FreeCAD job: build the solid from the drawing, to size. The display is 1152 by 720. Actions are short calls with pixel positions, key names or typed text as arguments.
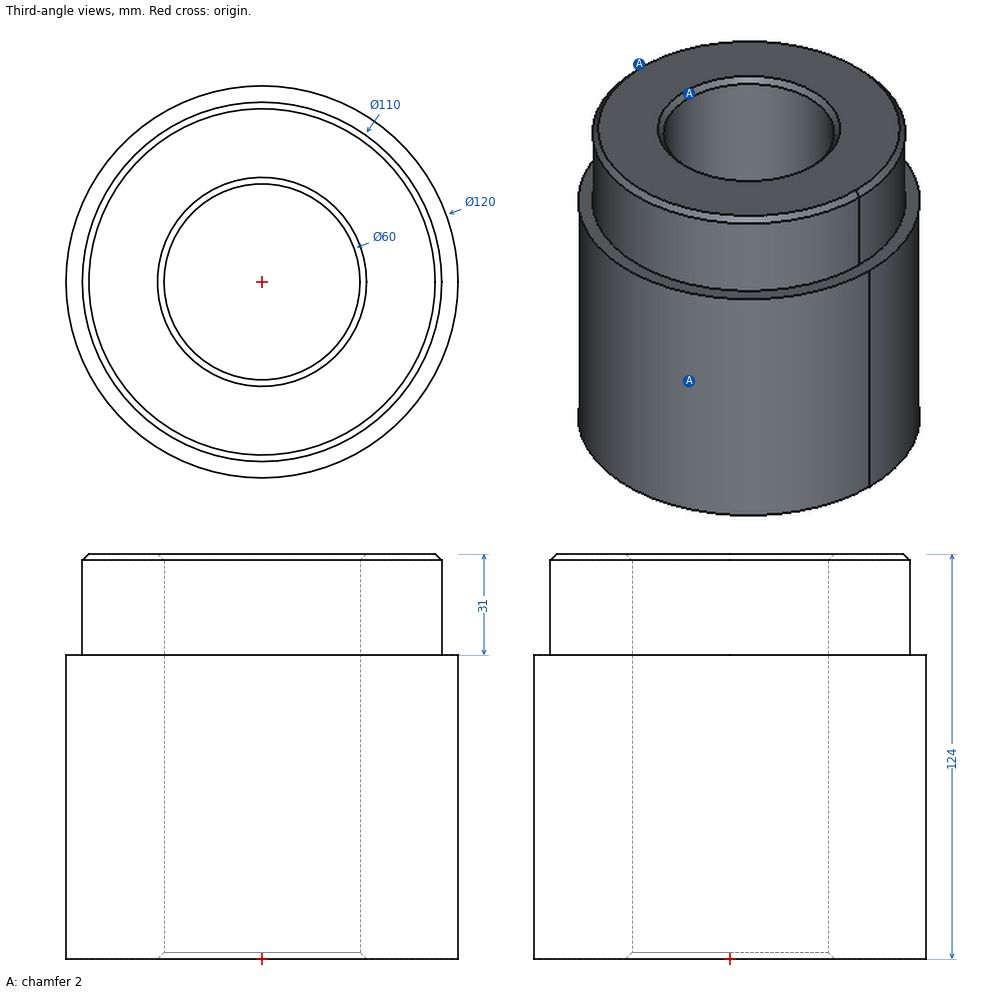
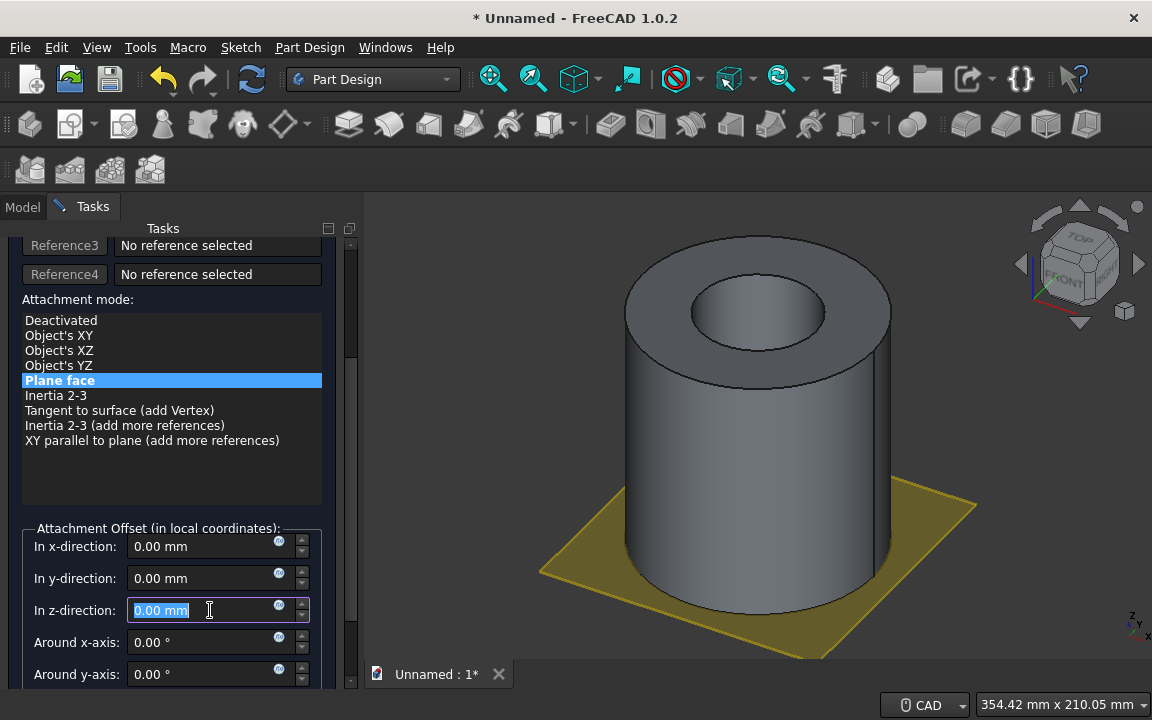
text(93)
key(Tab)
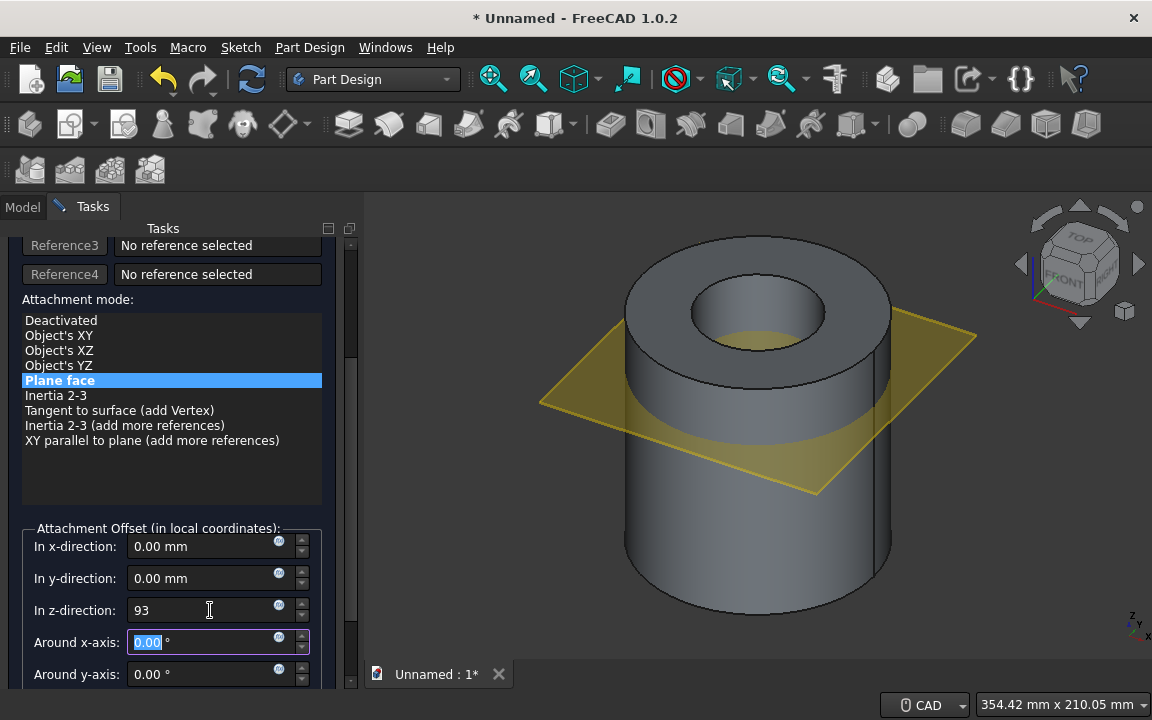
scroll(351, 463, up, 4)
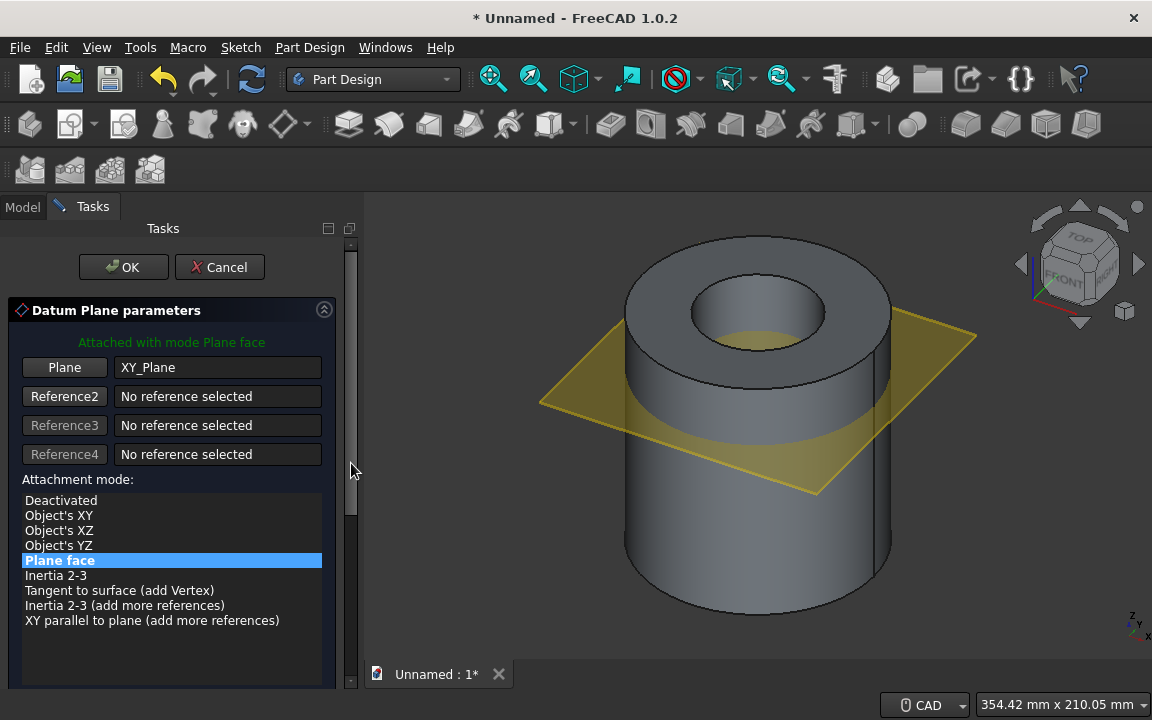
click(124, 267)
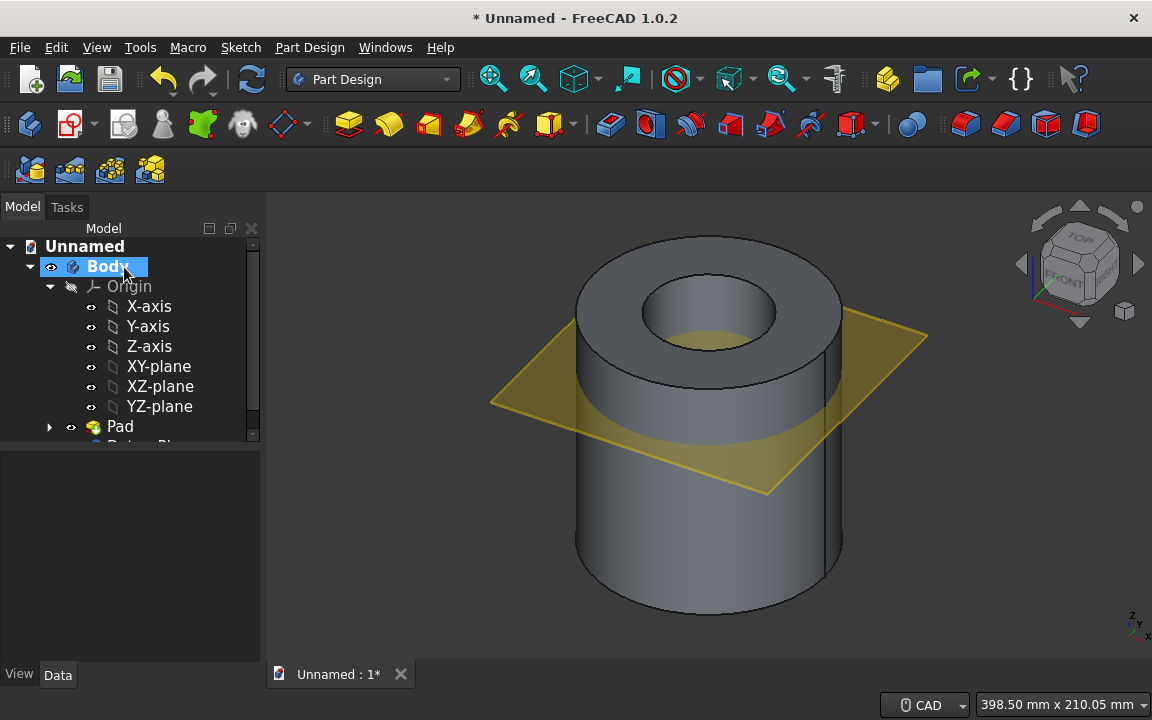
scroll(100, 342, down, 3)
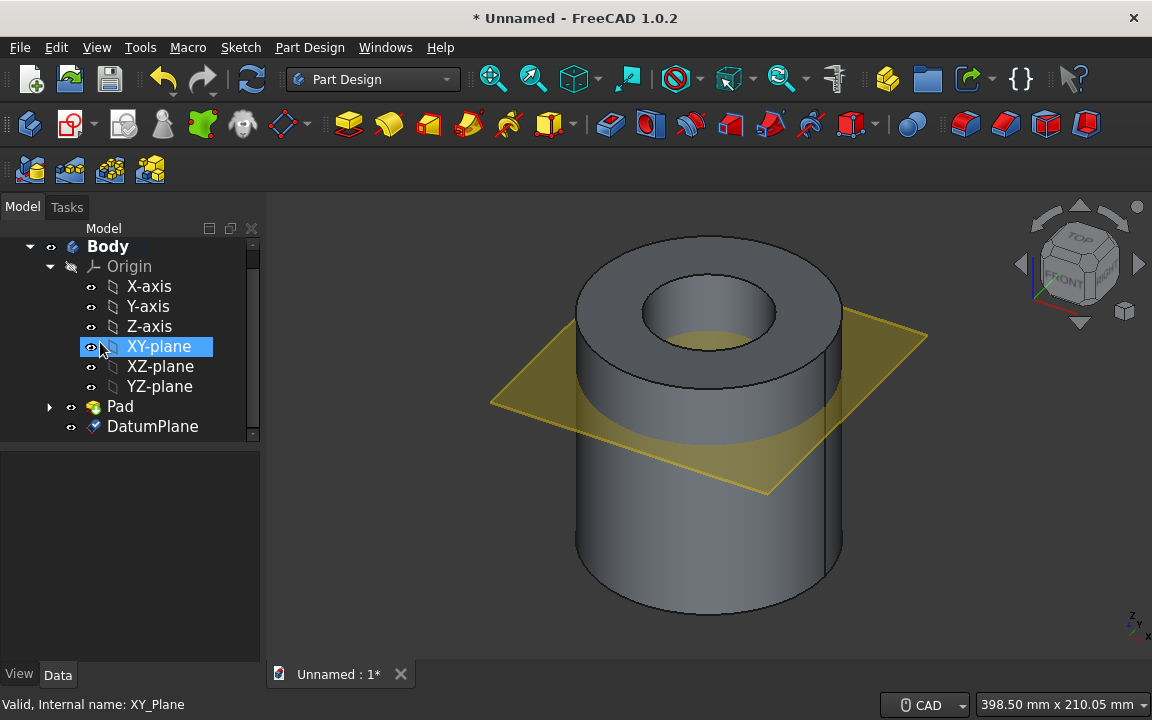
click(116, 427)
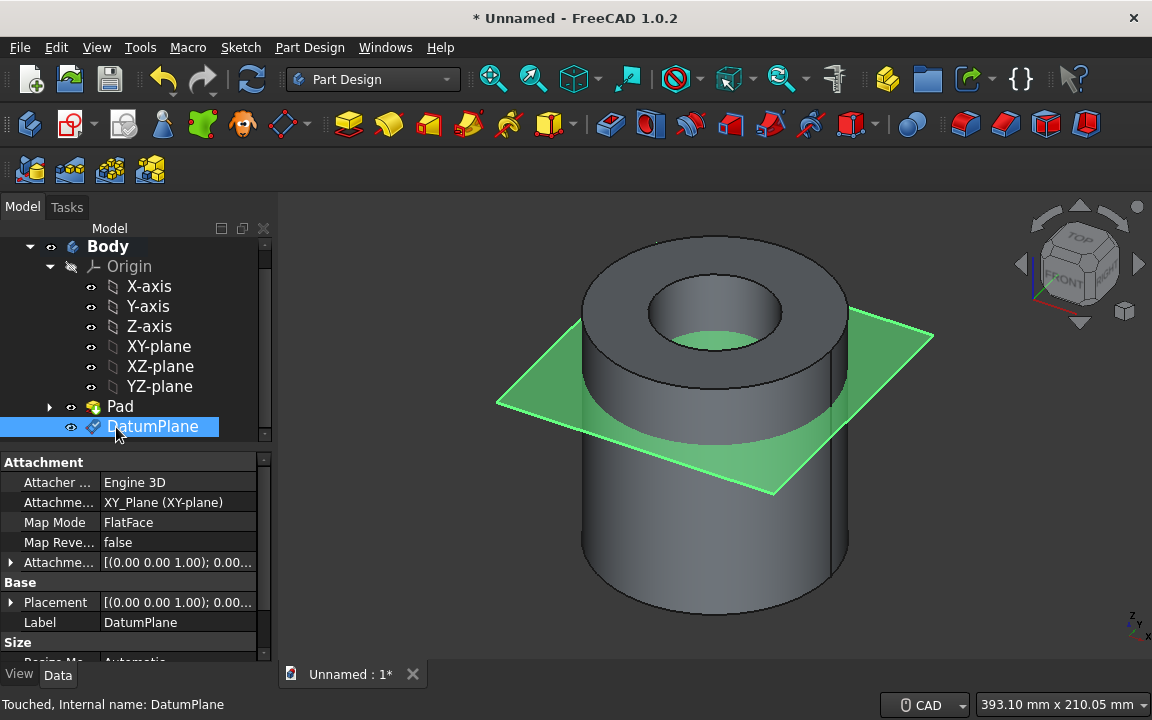
click(70, 124)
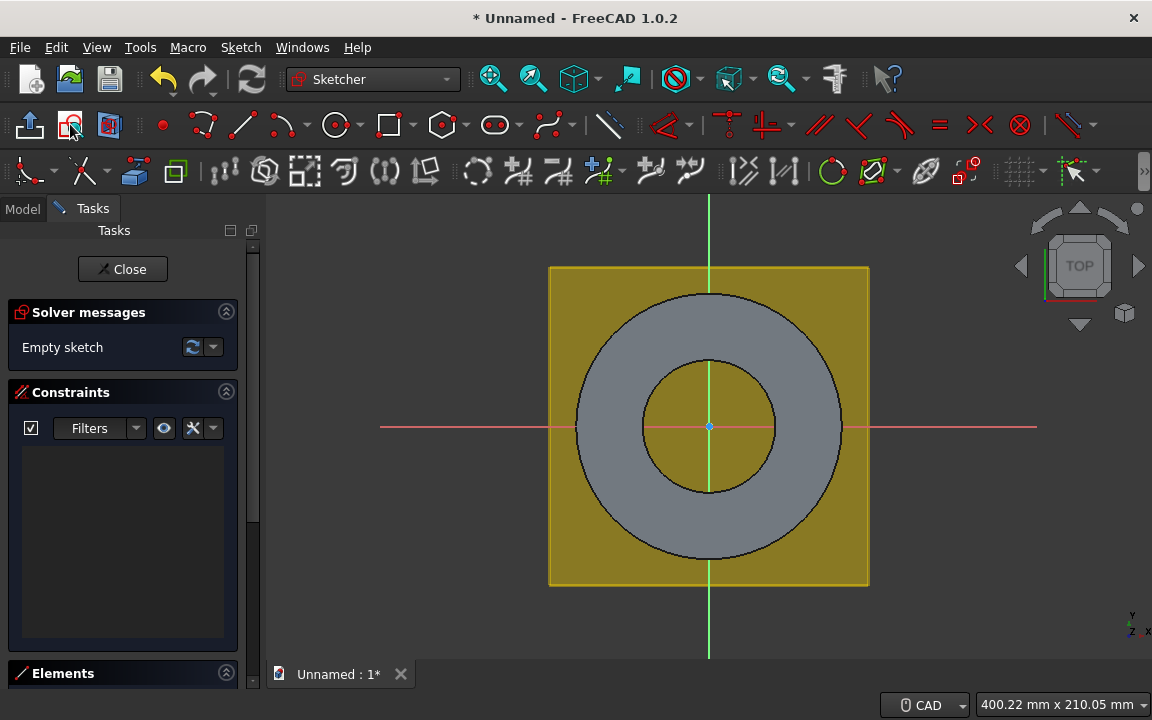
click(110, 126)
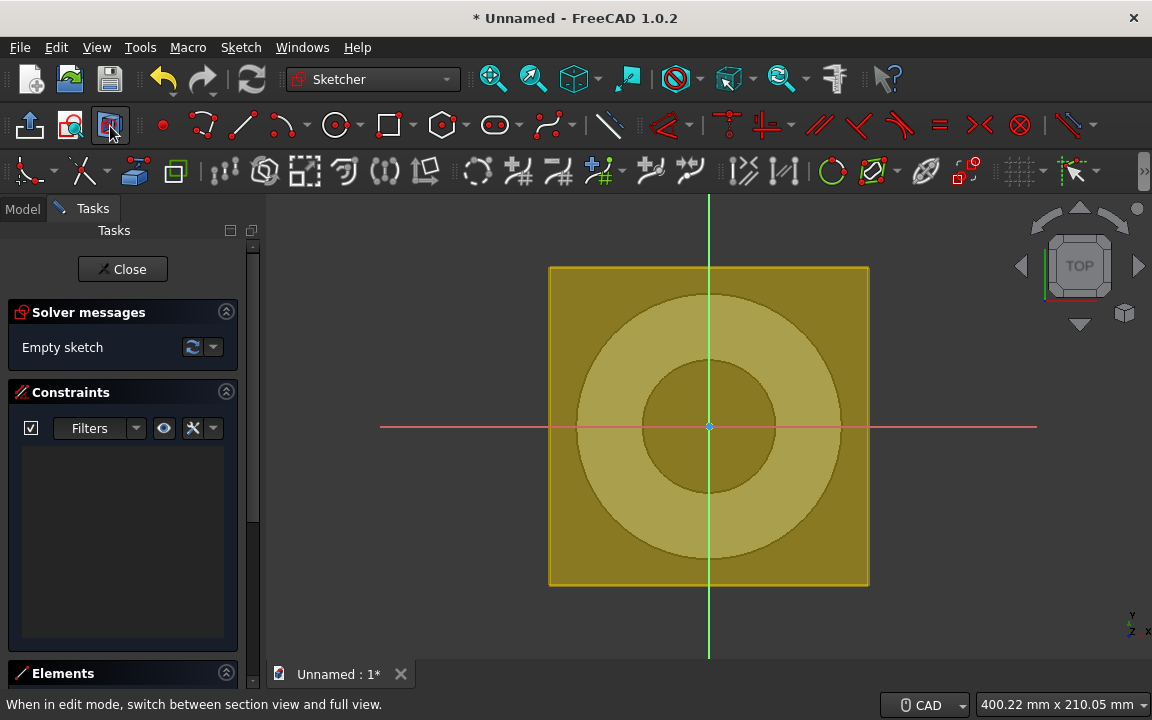
click(336, 126)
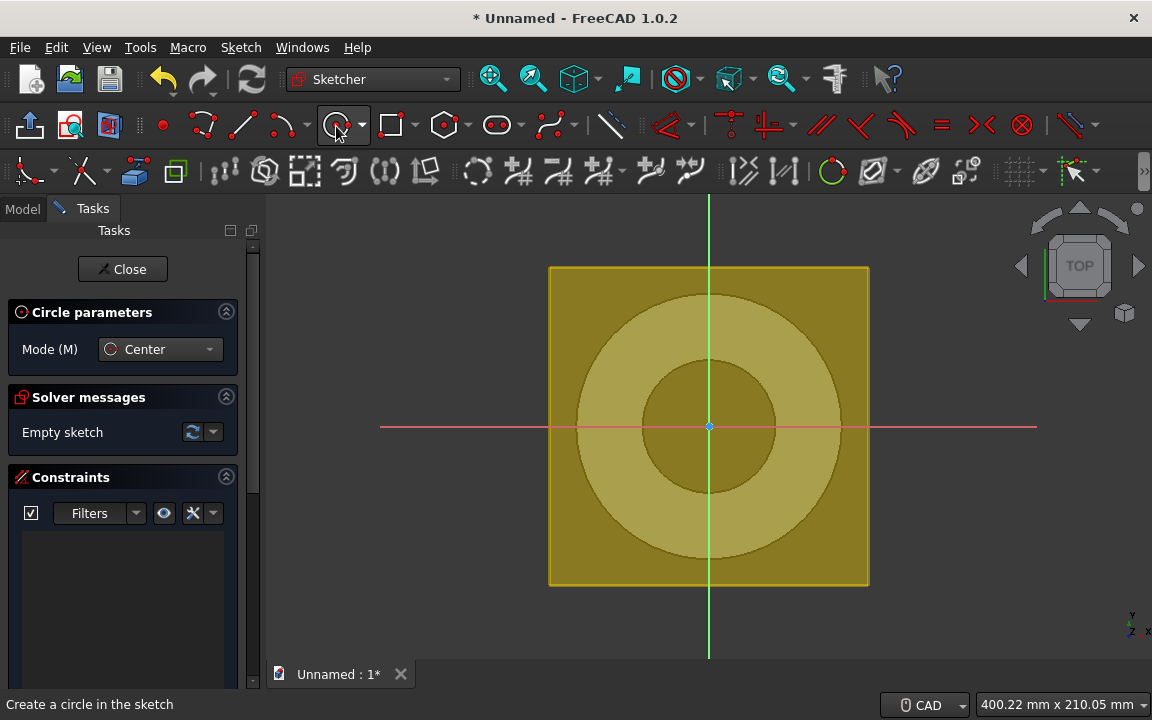
click(709, 426)
click(803, 333)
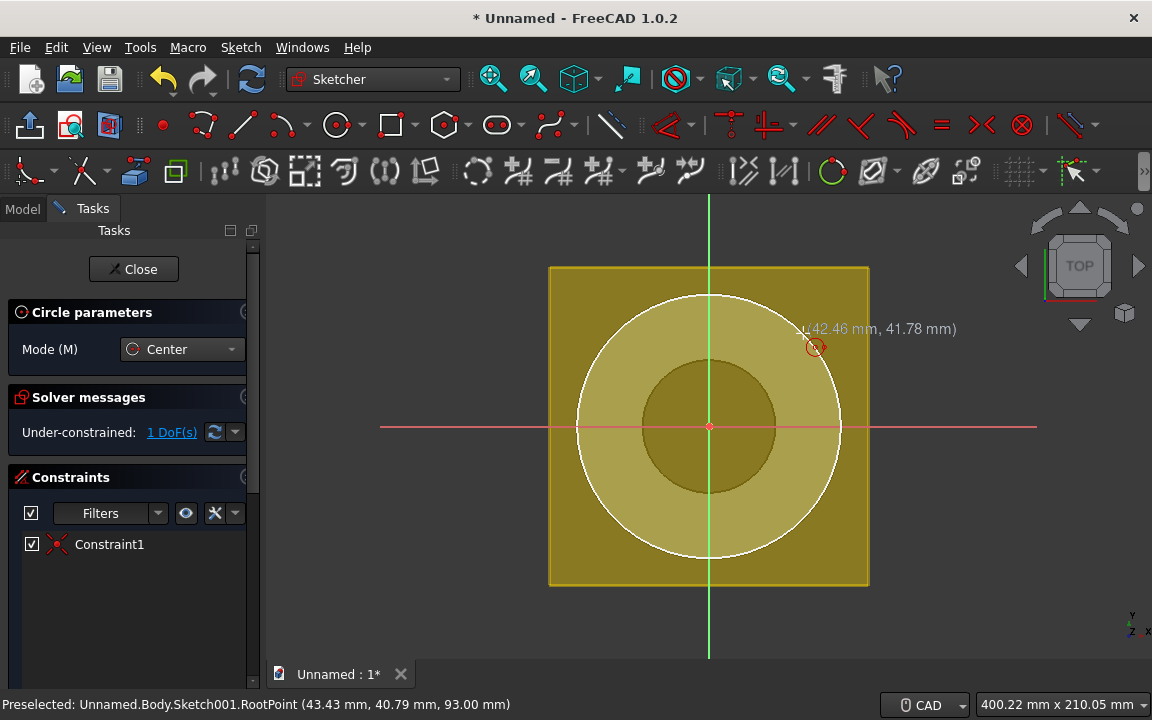
click(709, 426)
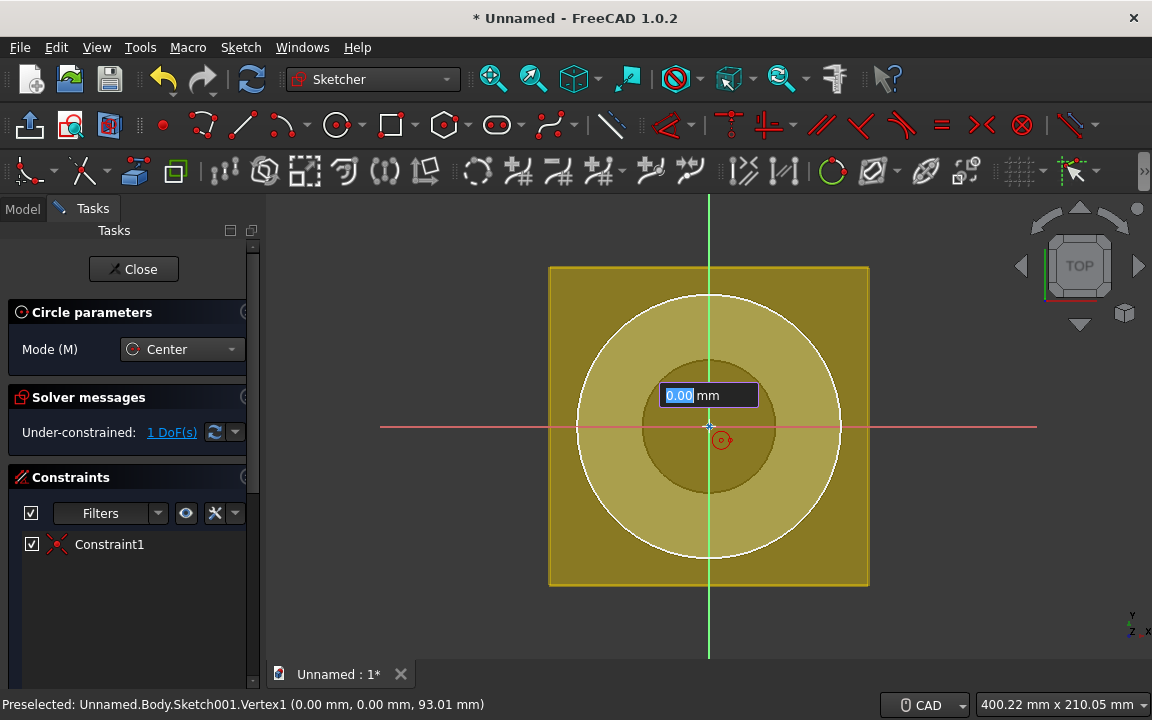
scroll(795, 340, up, 2)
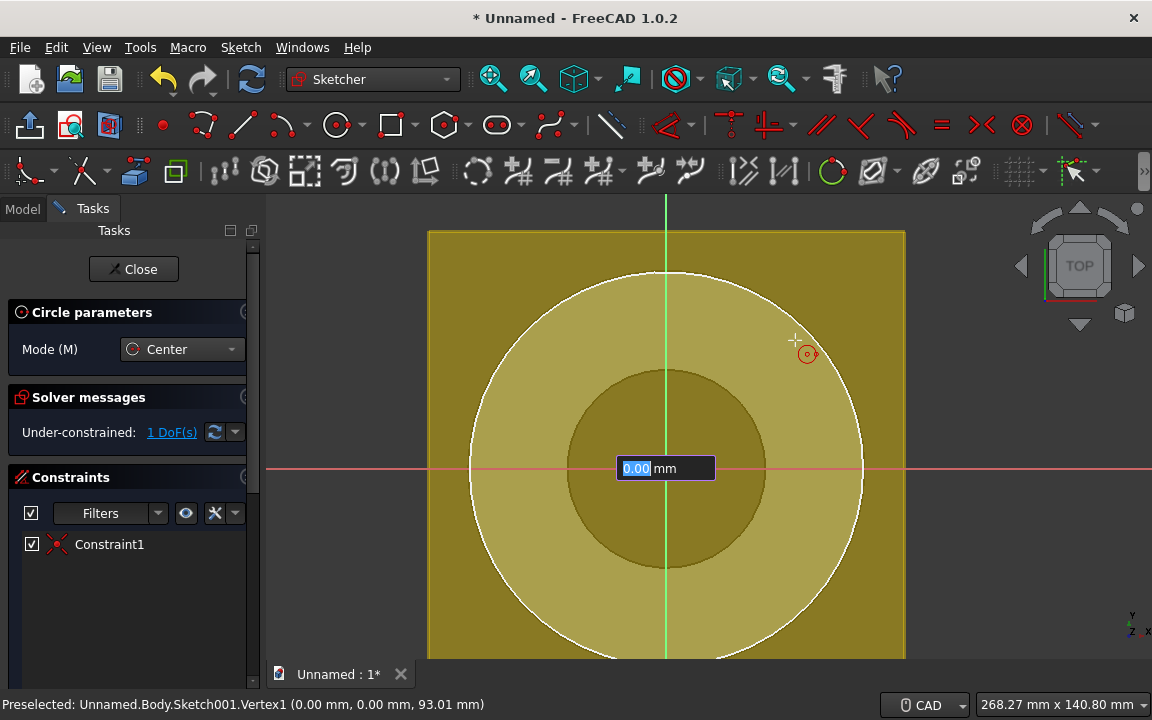
click(795, 340)
key(Escape)